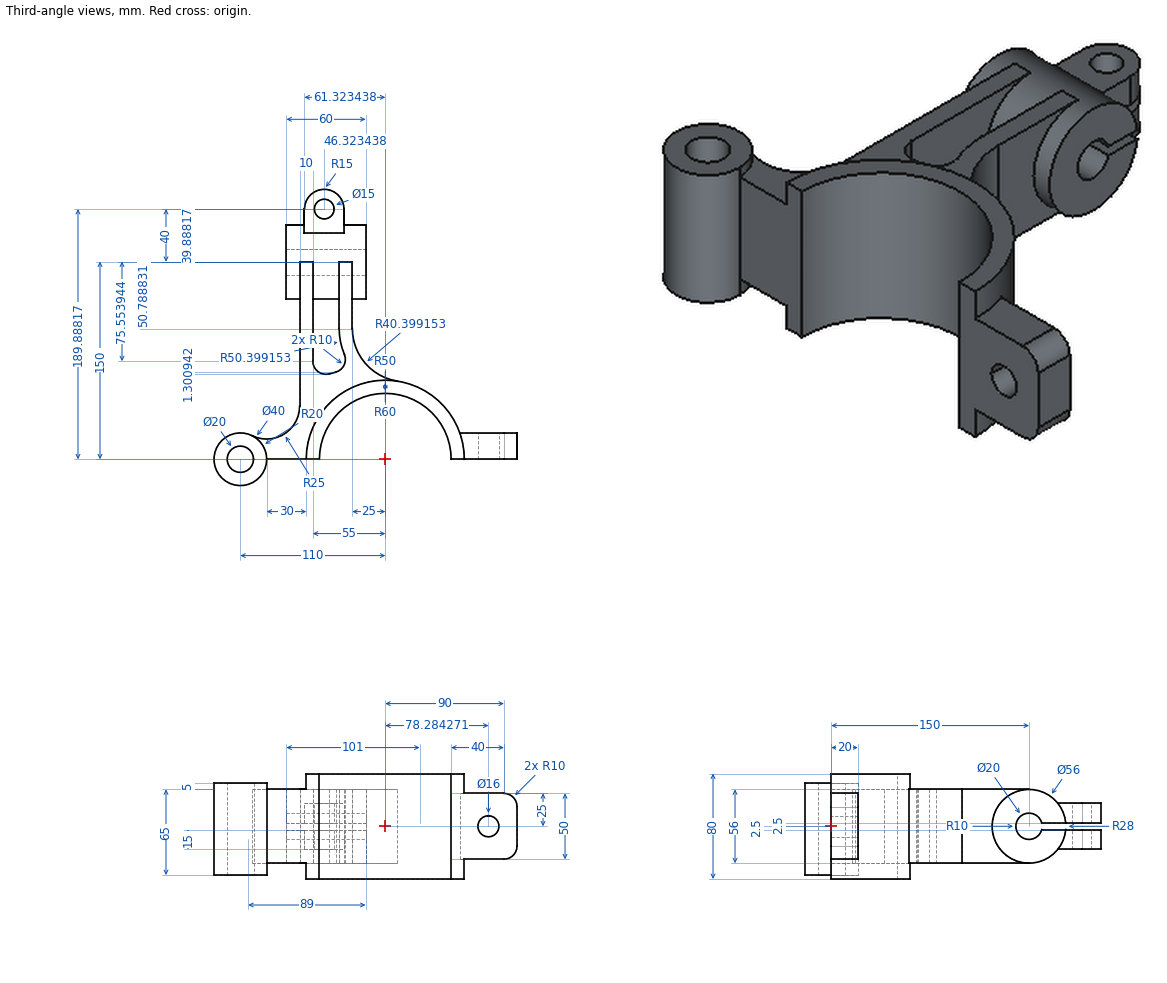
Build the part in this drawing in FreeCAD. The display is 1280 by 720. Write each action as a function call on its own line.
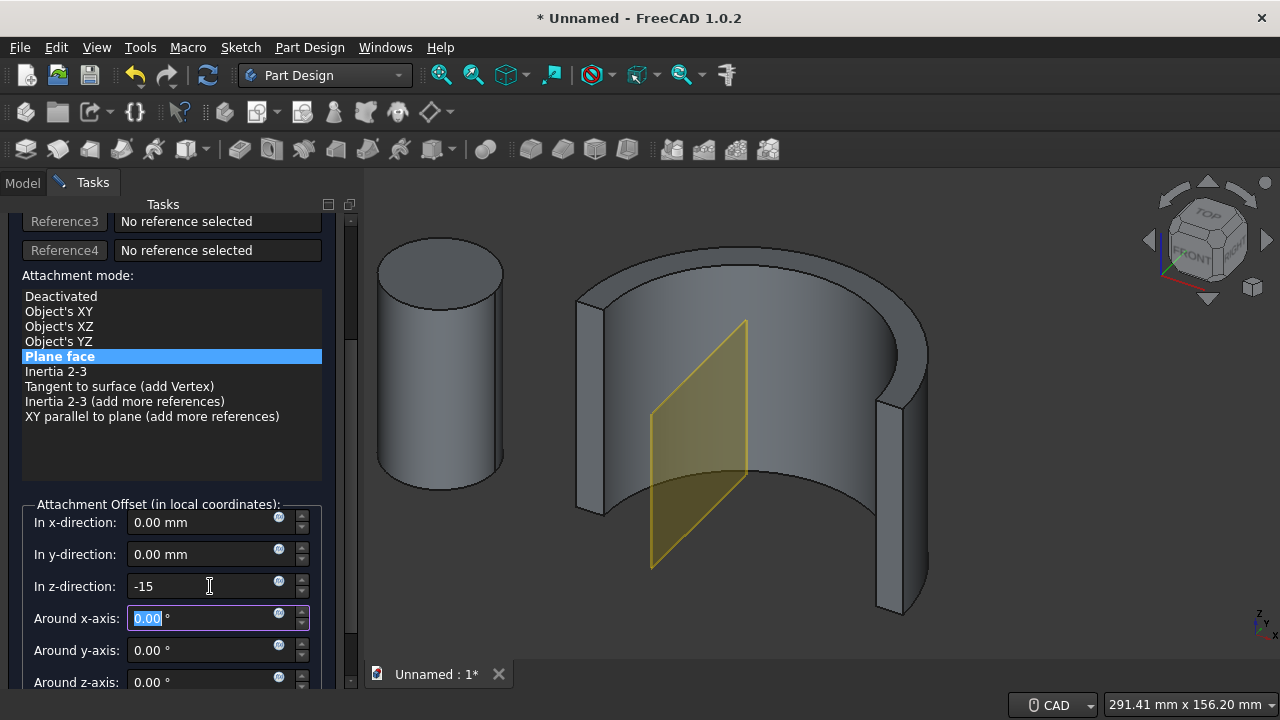
scroll(351, 451, up, 4)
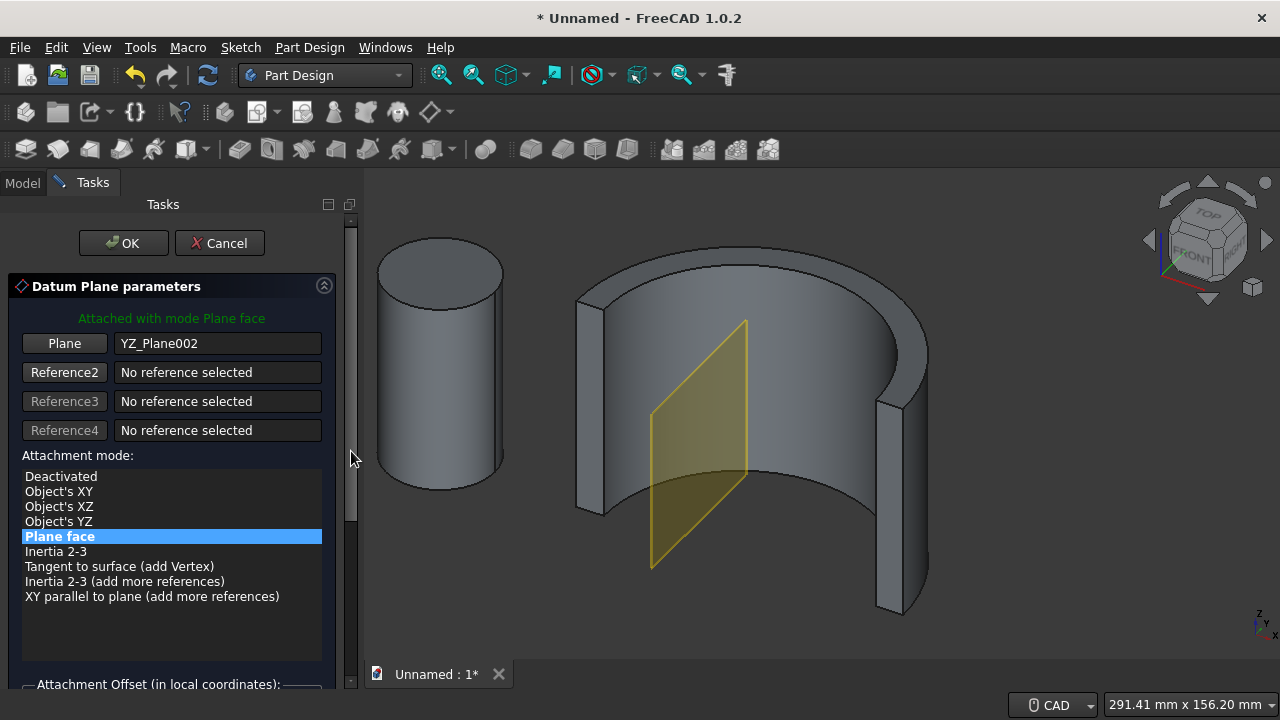
click(124, 243)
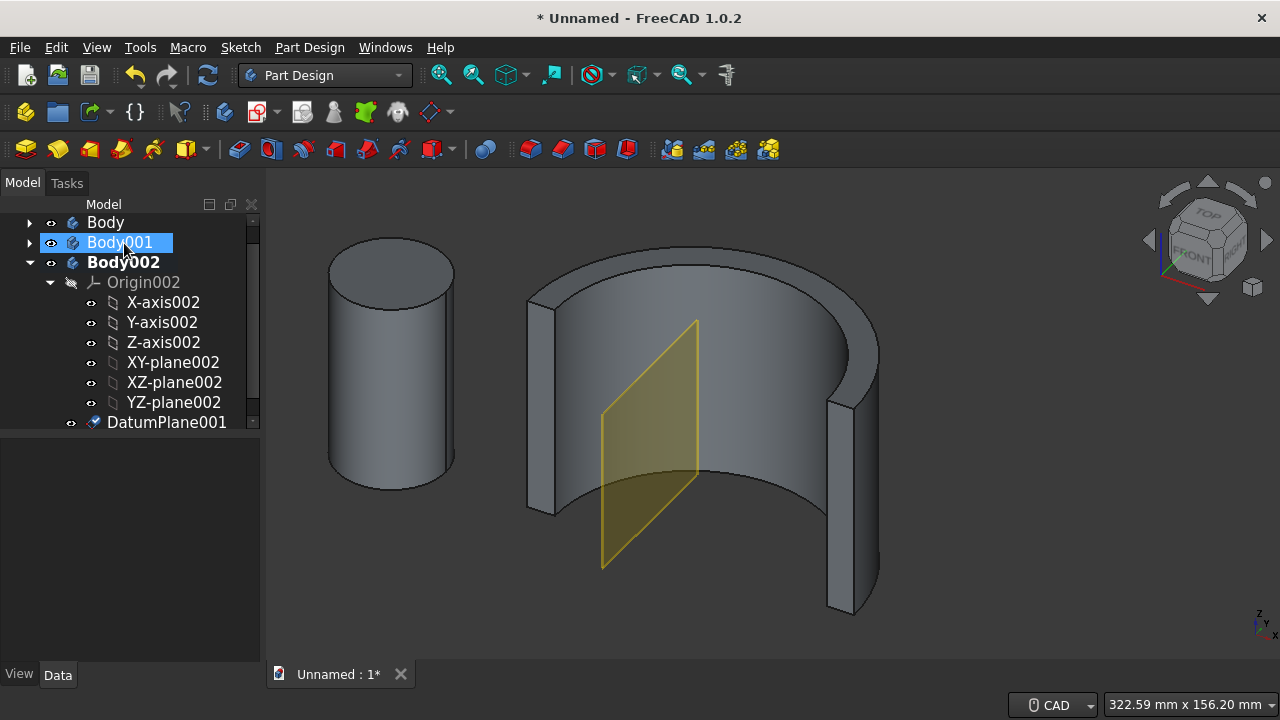
click(116, 423)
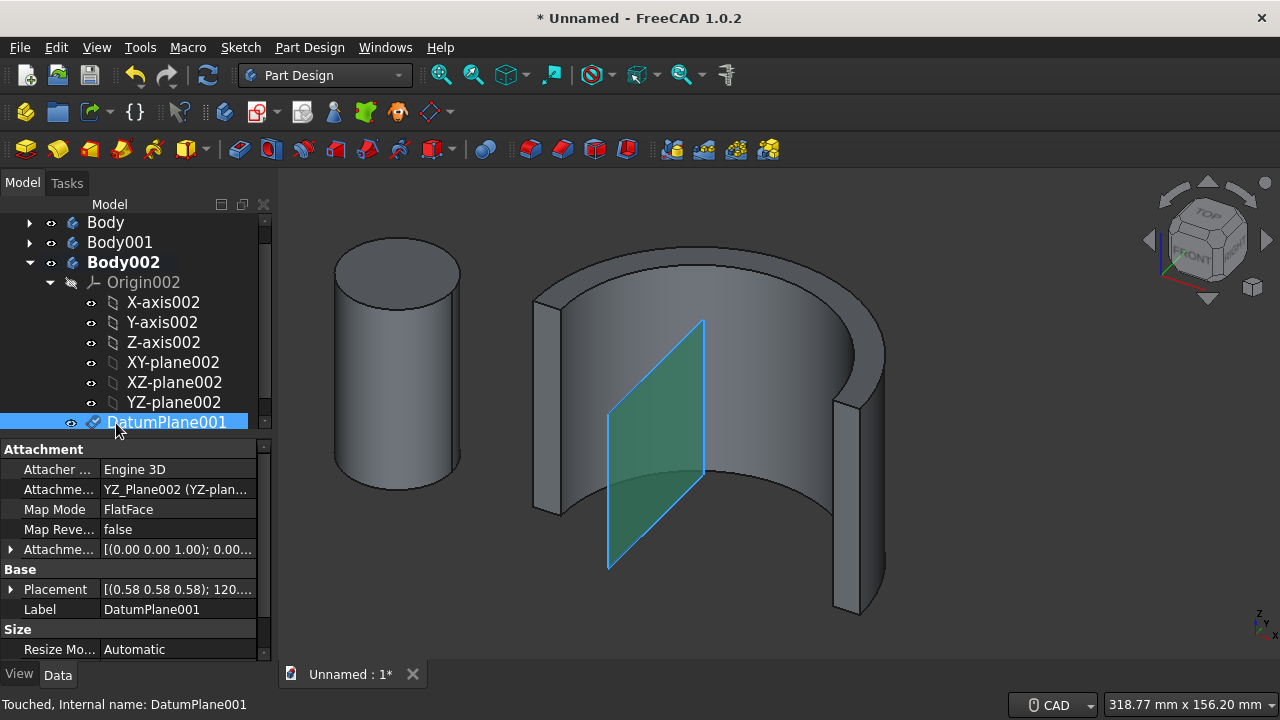
click(258, 112)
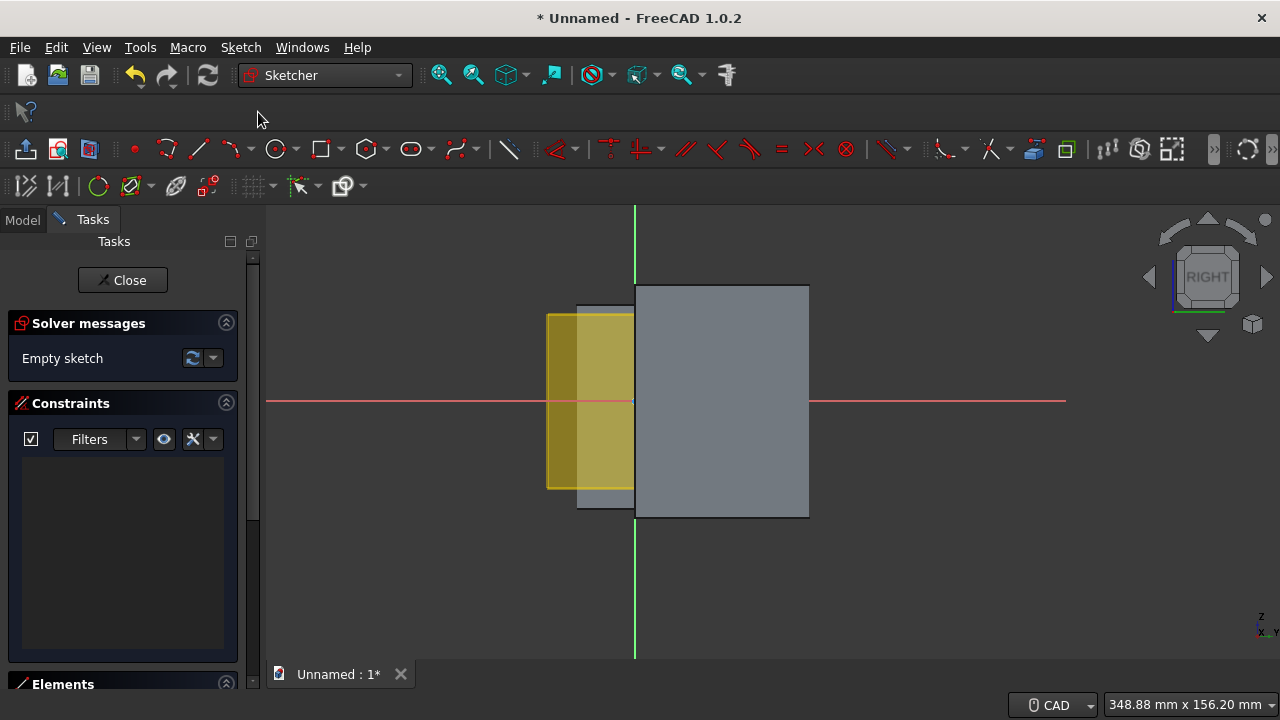
scroll(704, 432, down, 5)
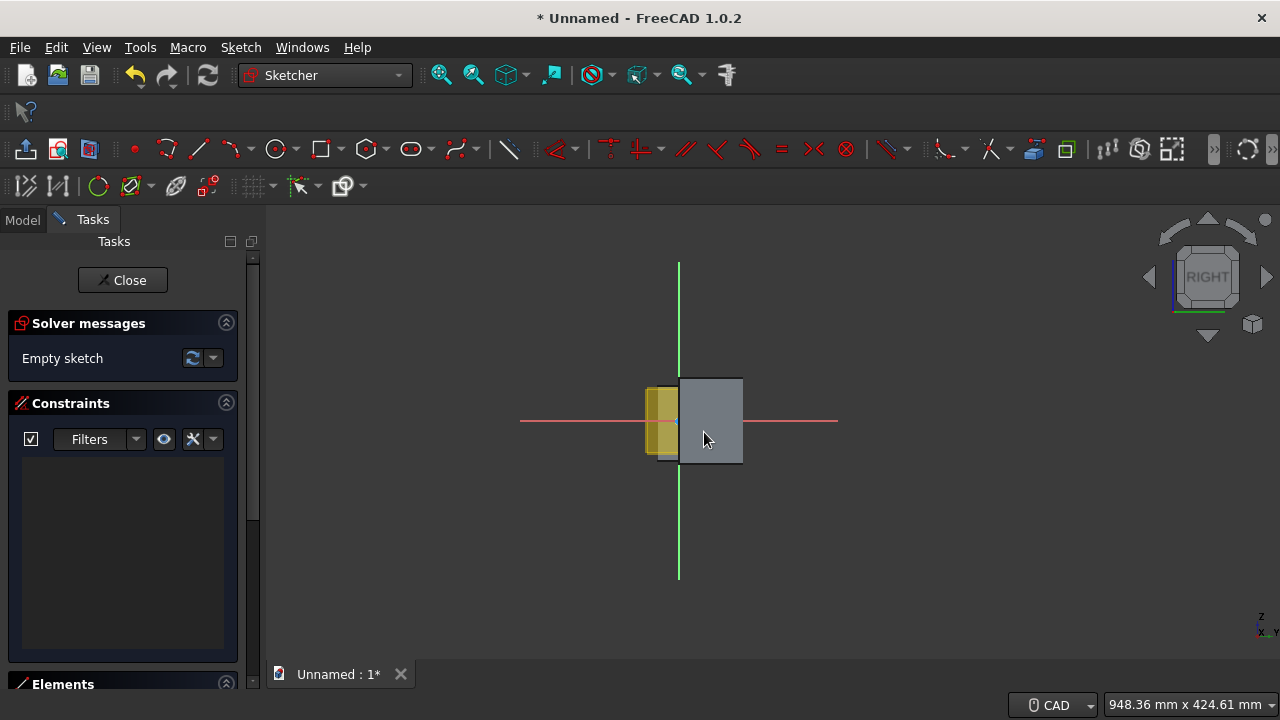
scroll(873, 418, up, 8)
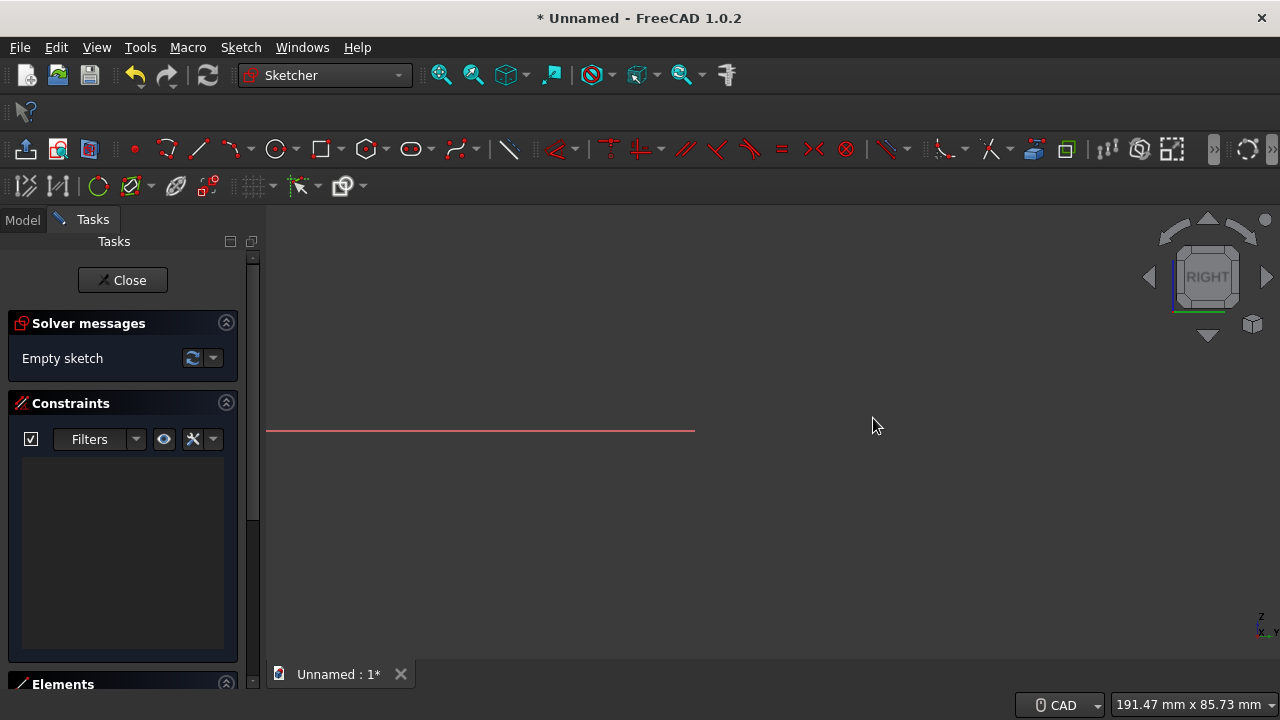
click(276, 150)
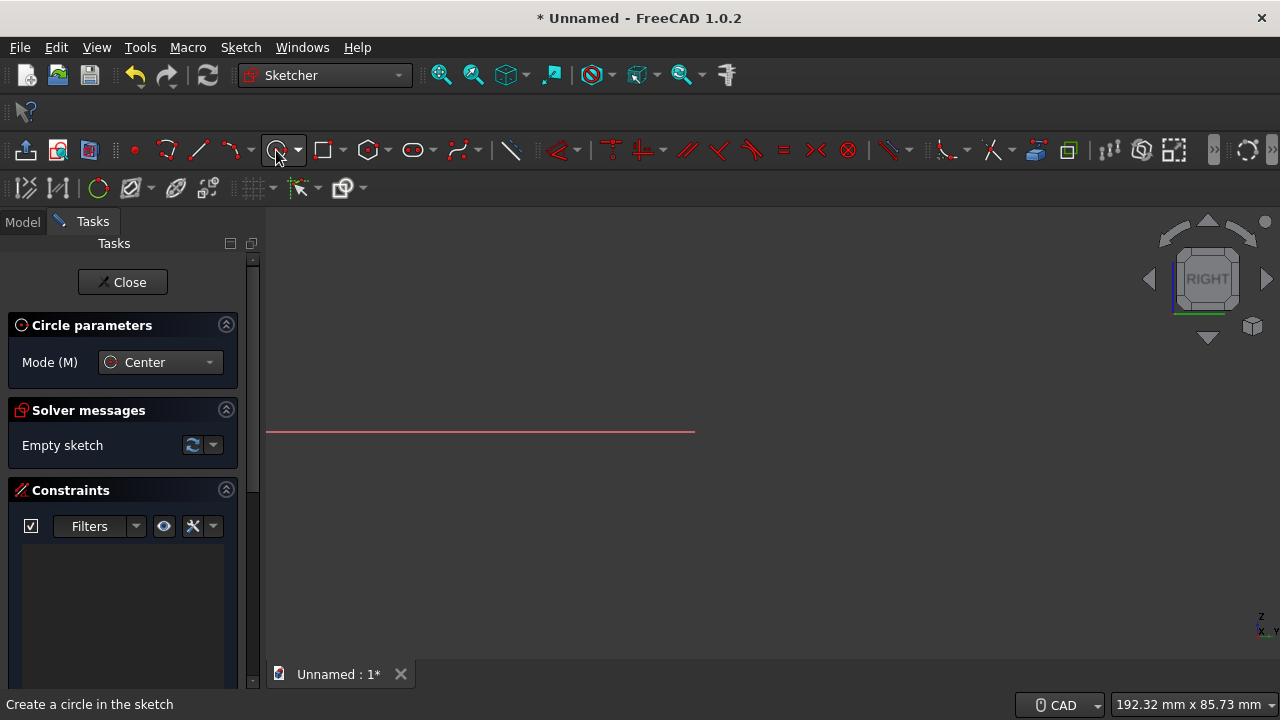
click(704, 432)
move(808, 328)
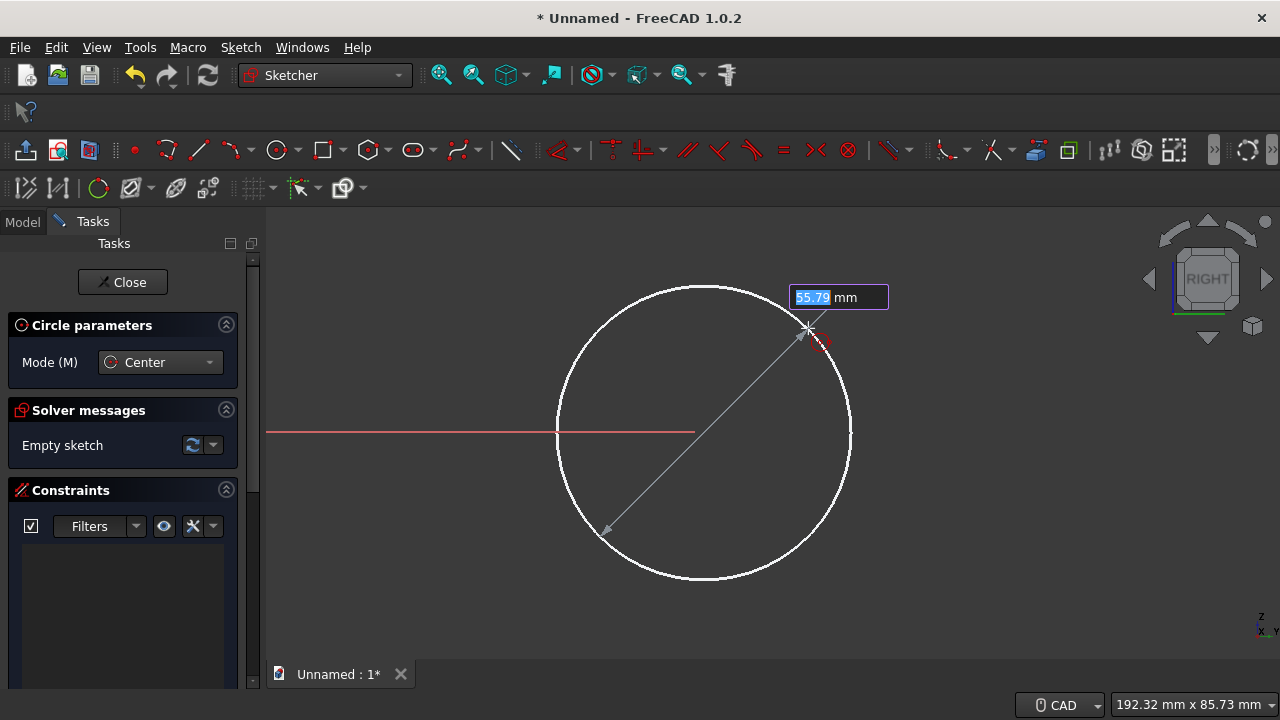
text(56)
key(Return)
key(Escape)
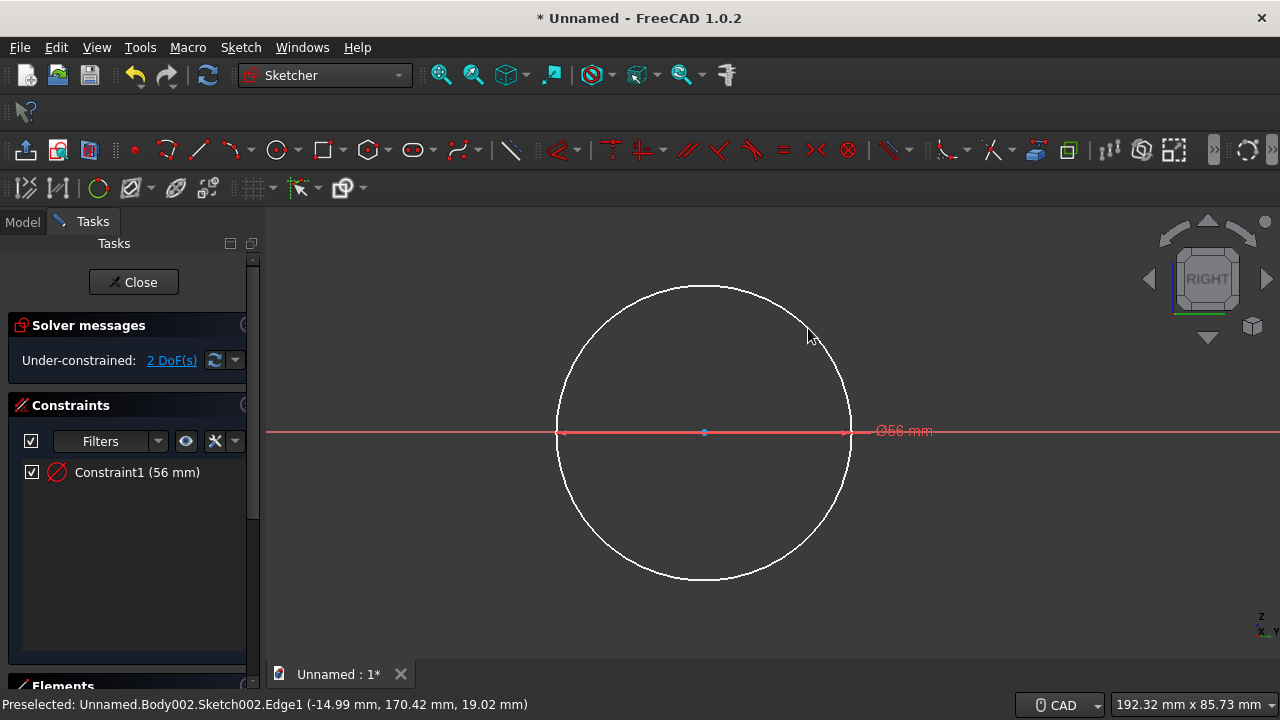
click(704, 433)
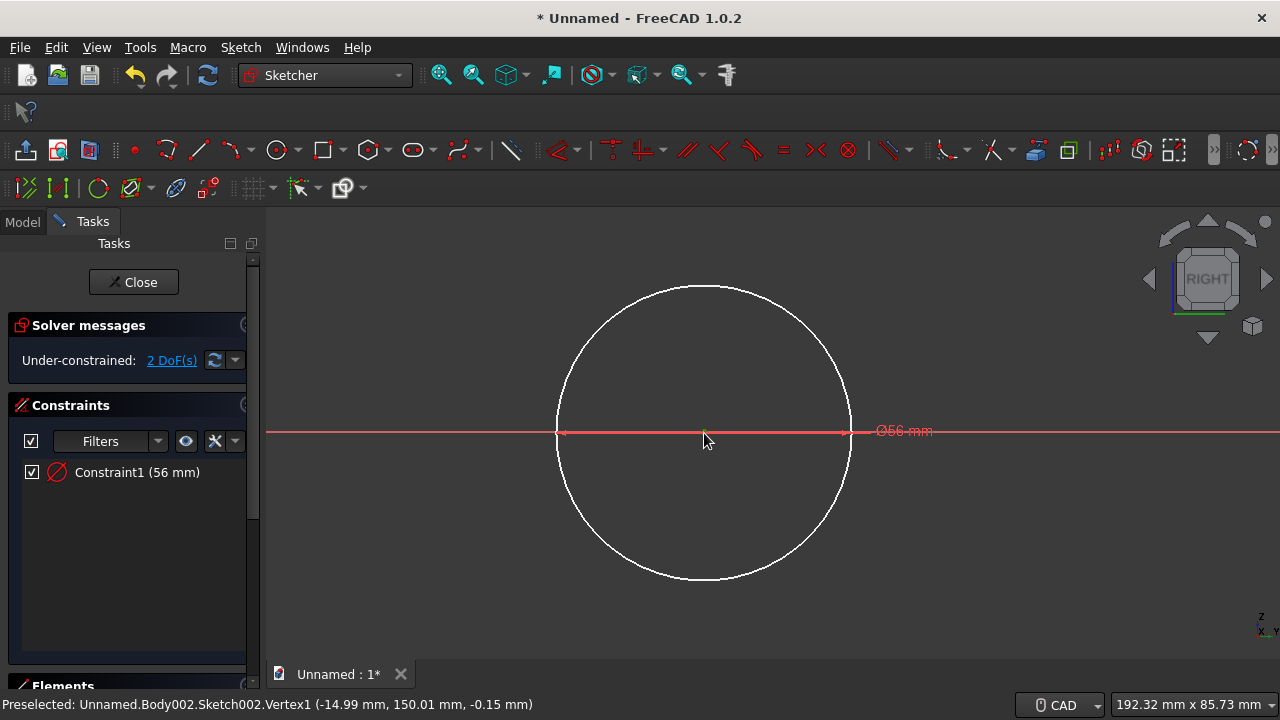
click(353, 432)